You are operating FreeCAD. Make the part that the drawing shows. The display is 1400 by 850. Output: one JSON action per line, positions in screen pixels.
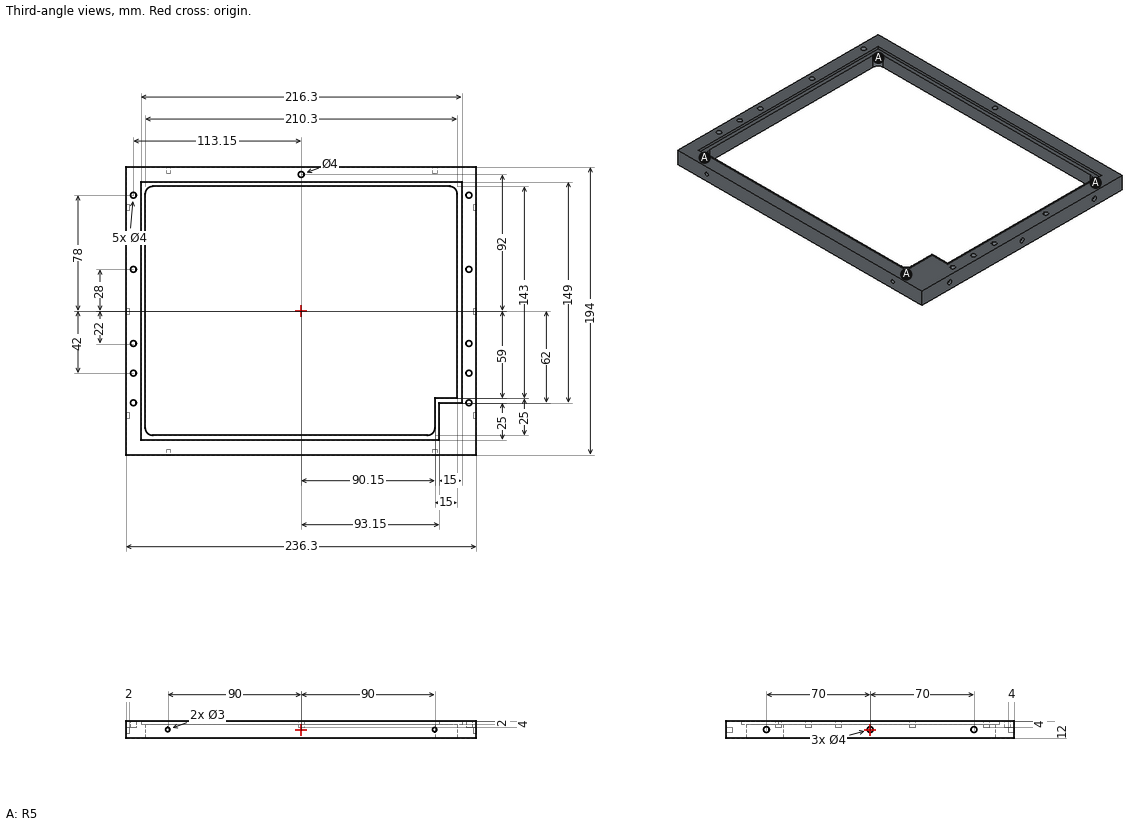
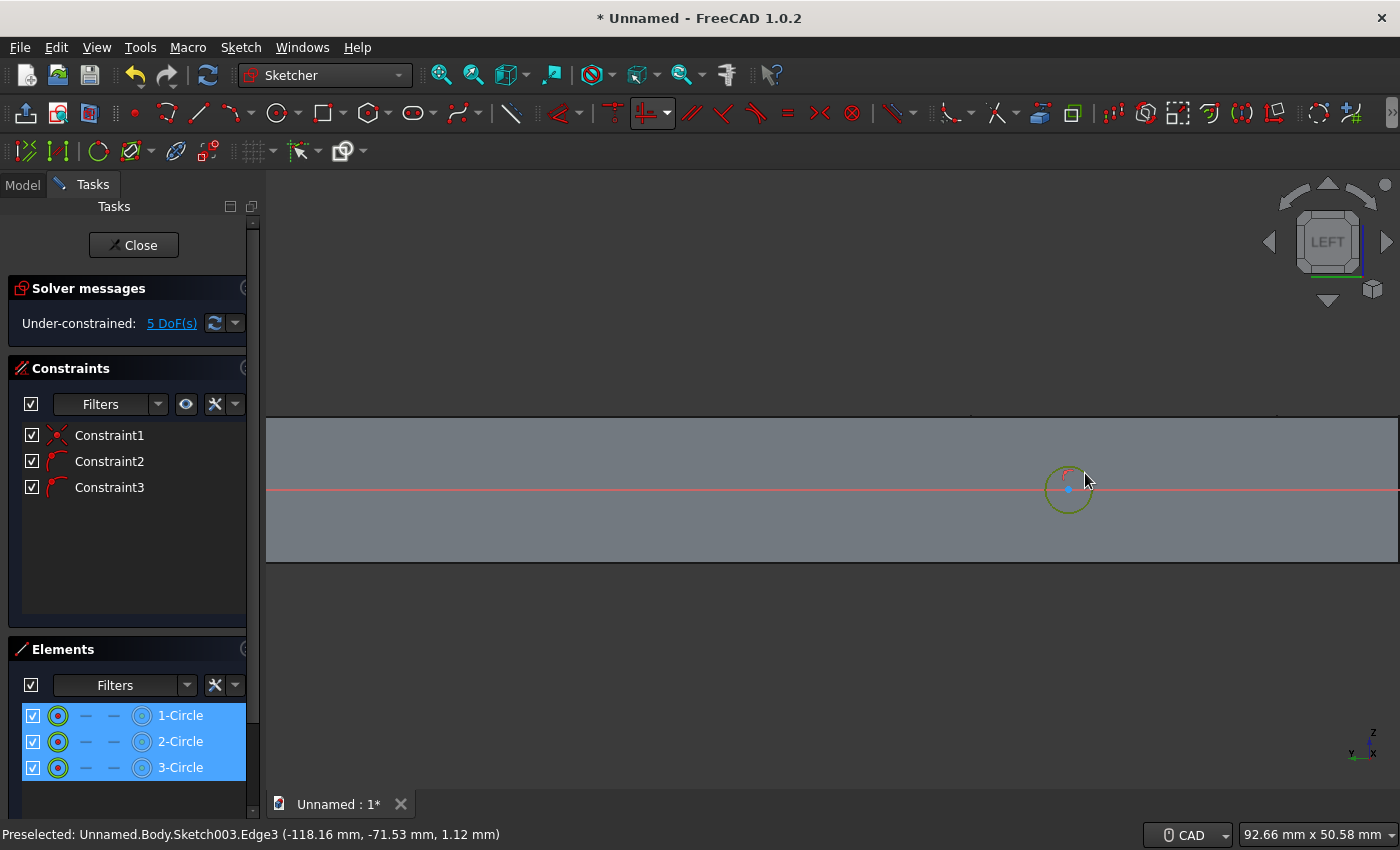
{"action": "left_click", "coordinate": [788, 114]}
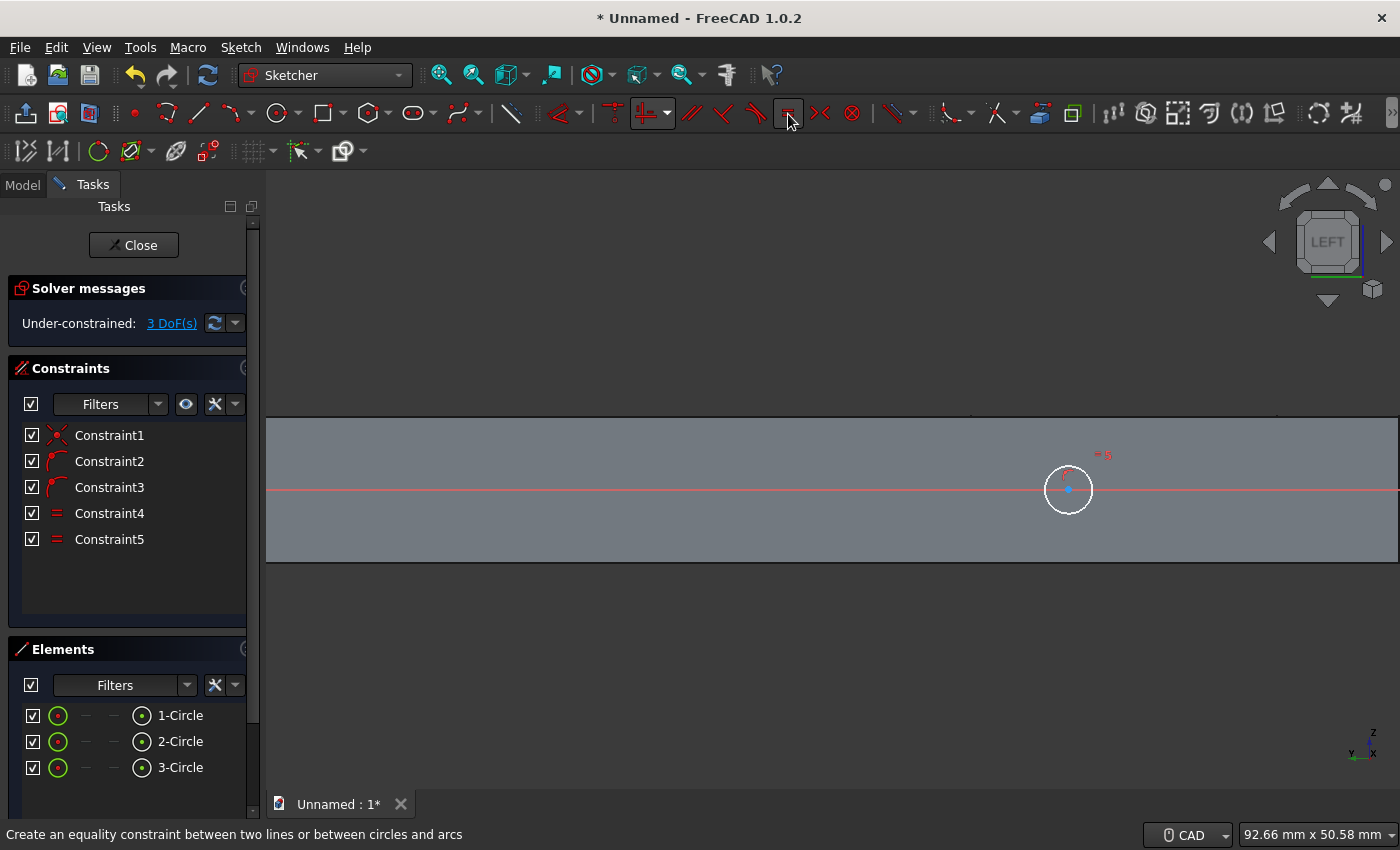
{"action": "left_click", "coordinate": [558, 114]}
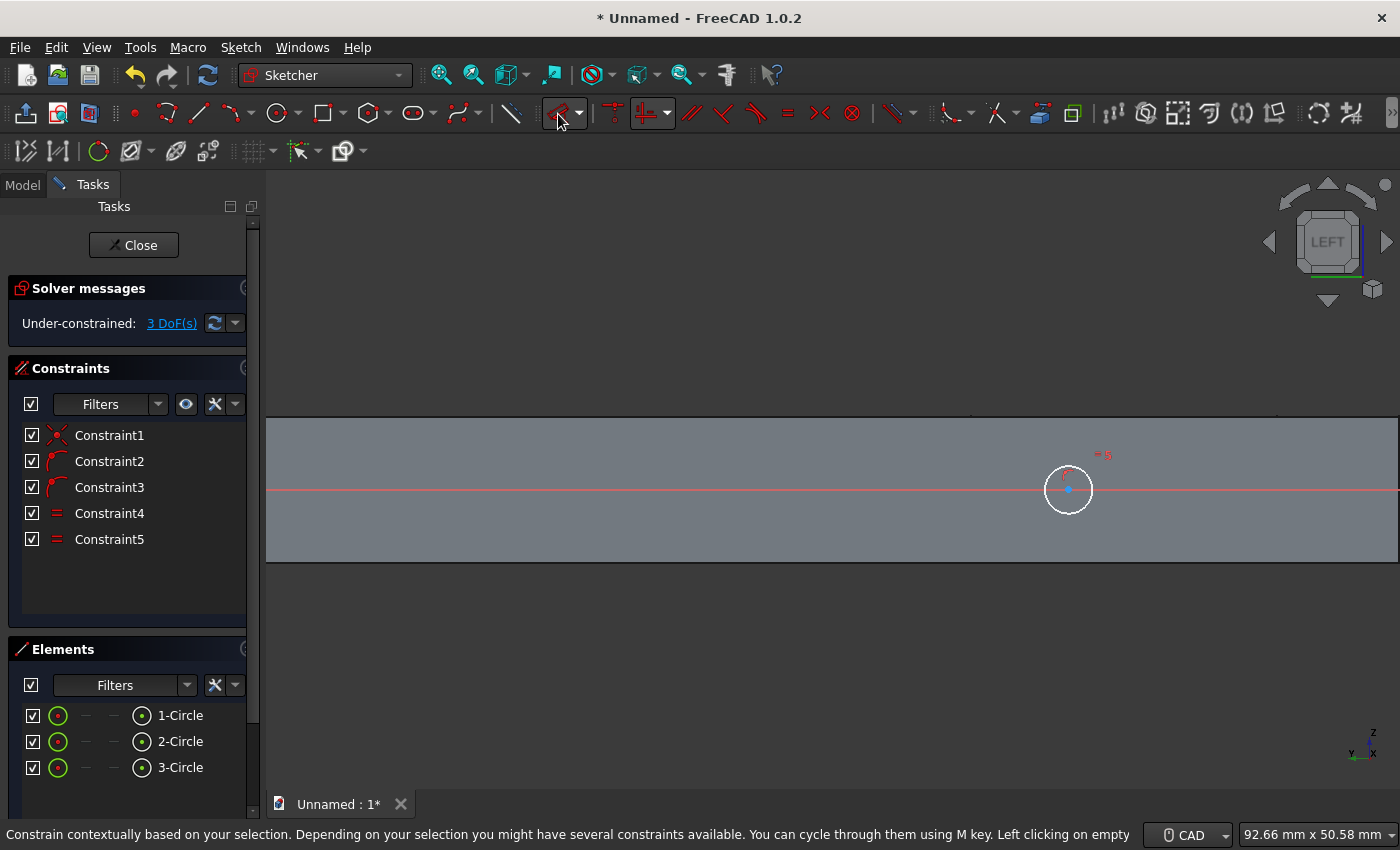
{"action": "scroll", "coordinate": [1086, 473], "scroll_direction": "down", "scroll_amount": 5}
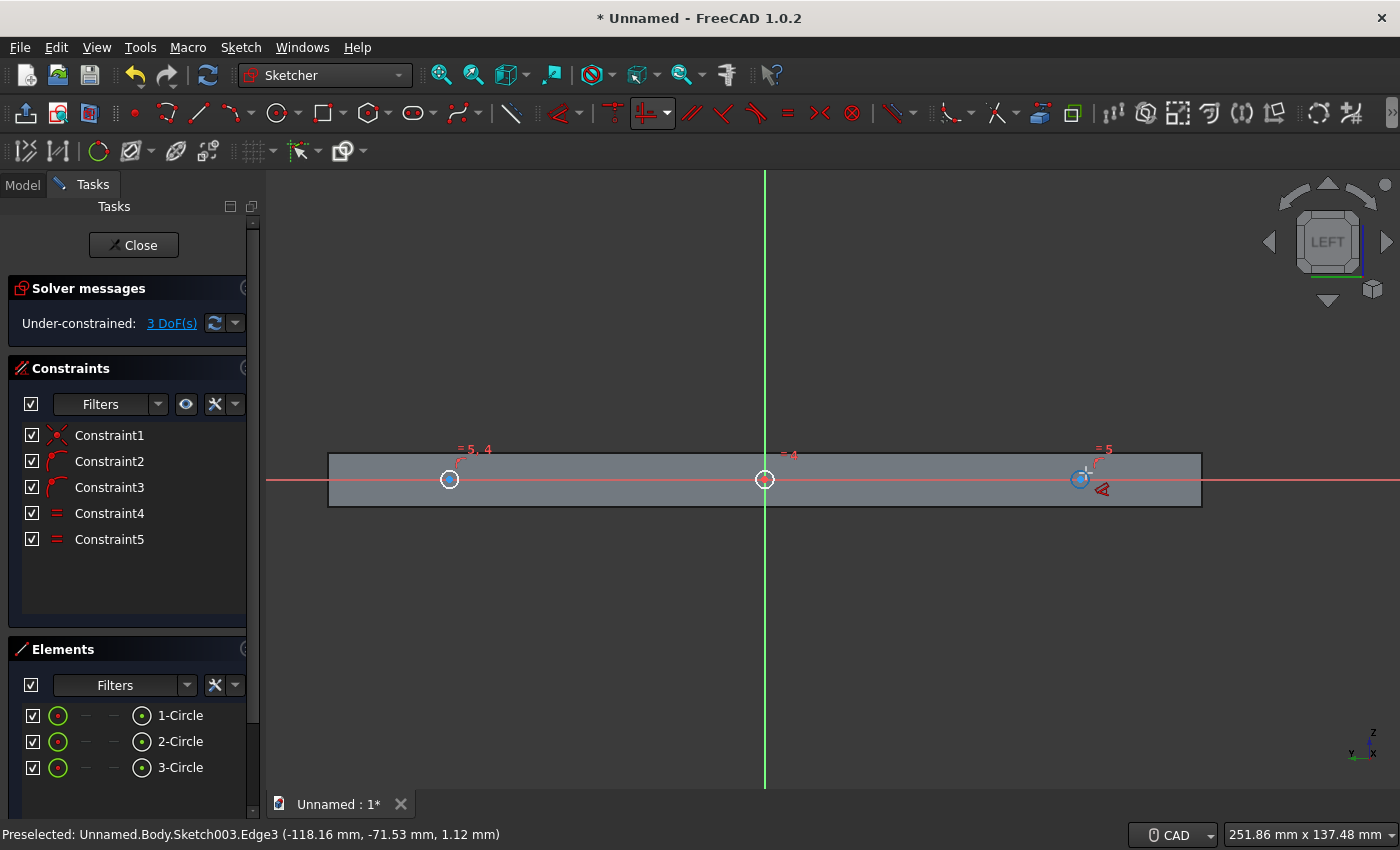
{"action": "scroll", "coordinate": [771, 473], "scroll_direction": "up", "scroll_amount": 5}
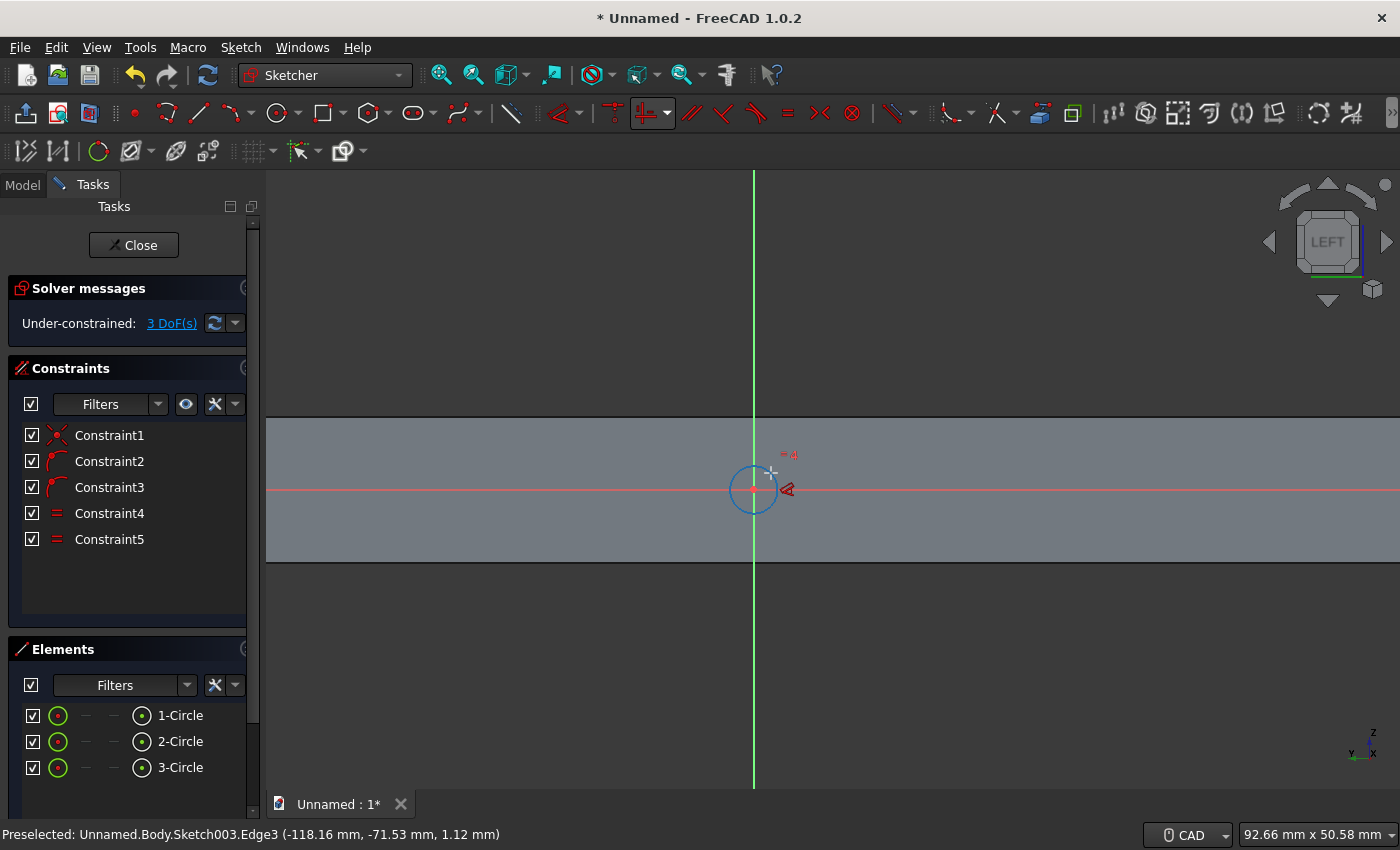
{"action": "left_click", "coordinate": [771, 473]}
{"action": "left_click", "coordinate": [794, 451]}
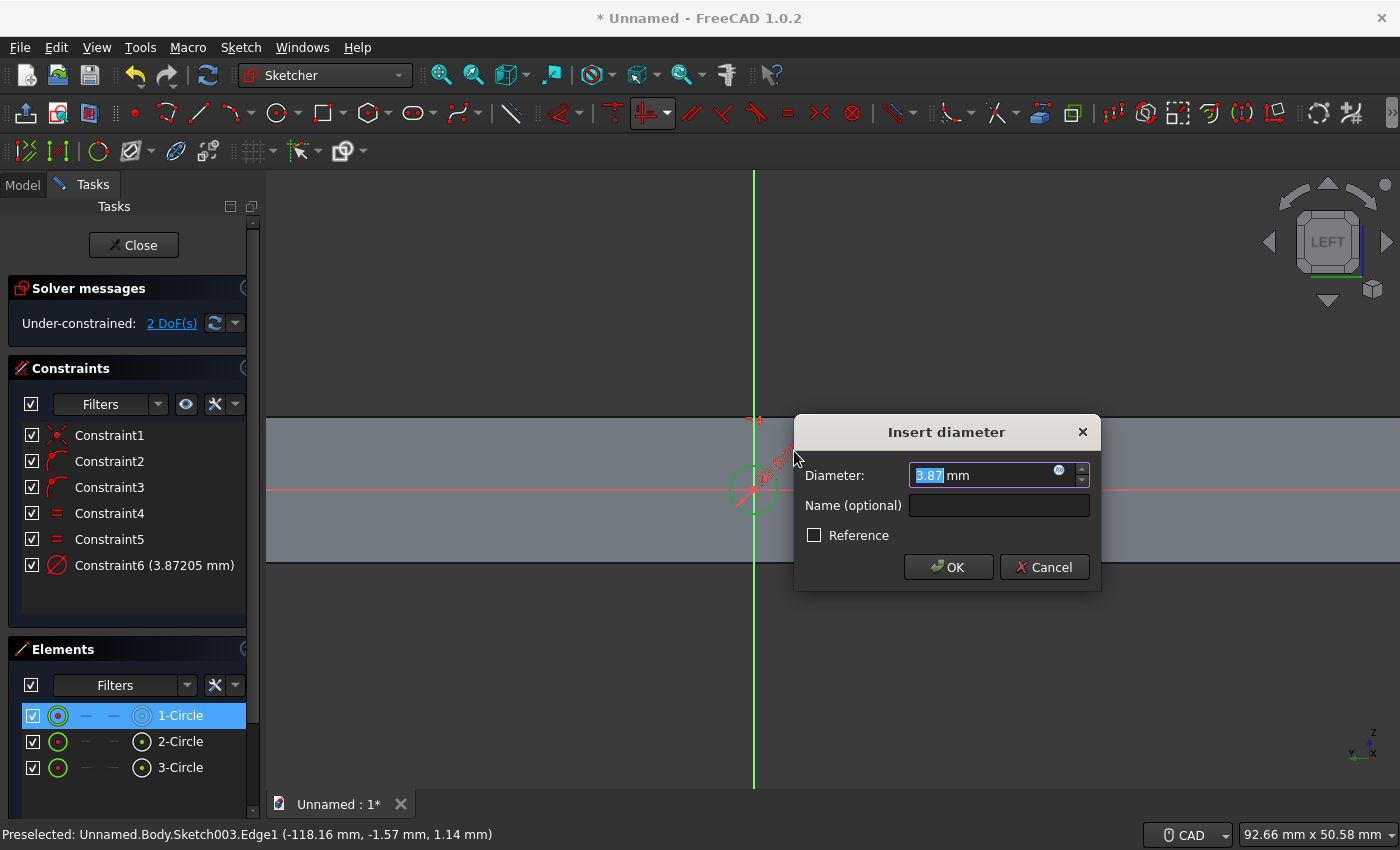
{"action": "type", "text": "4"}
{"action": "key", "text": "Return"}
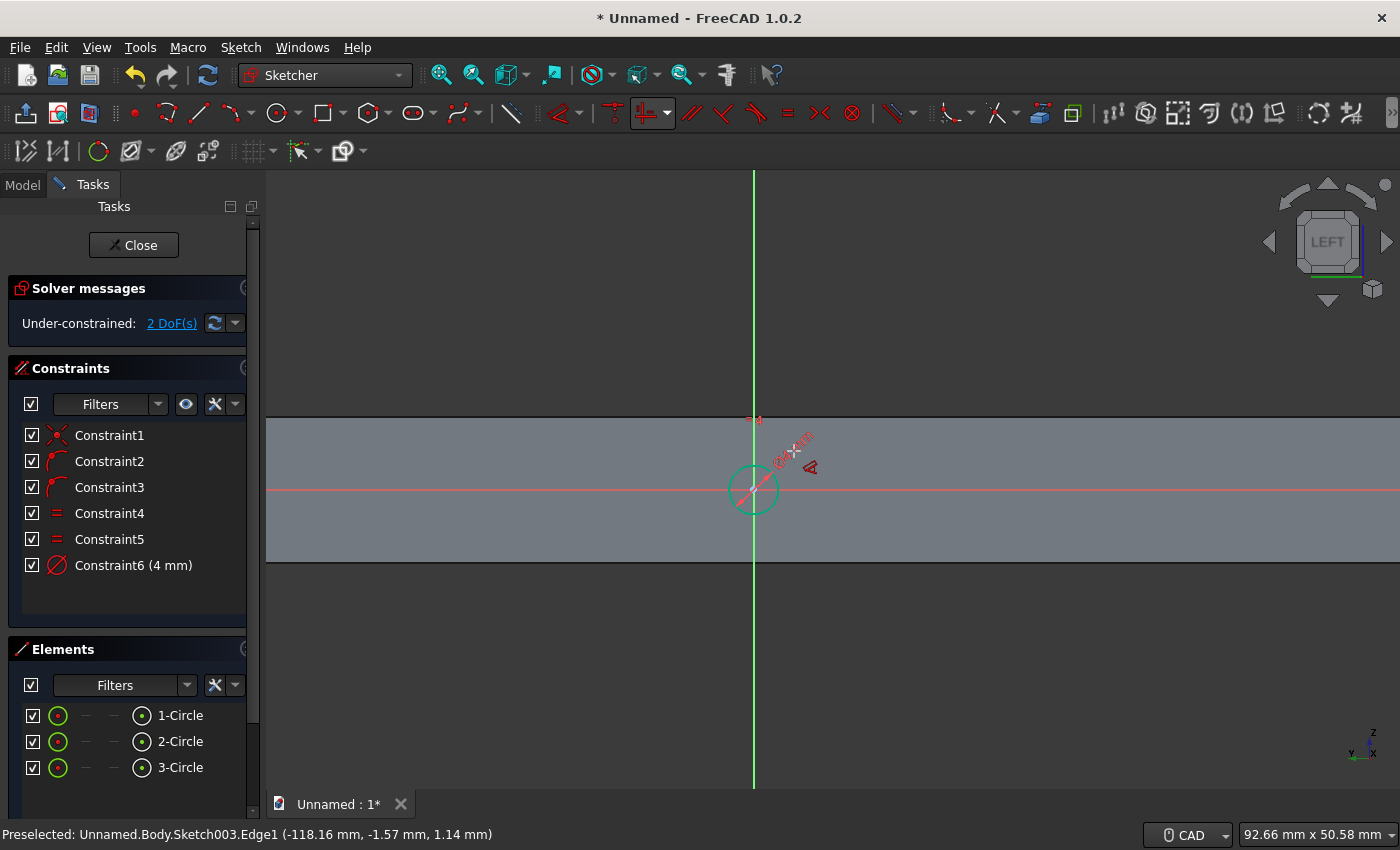
{"action": "scroll", "coordinate": [771, 473], "scroll_direction": "down", "scroll_amount": 5}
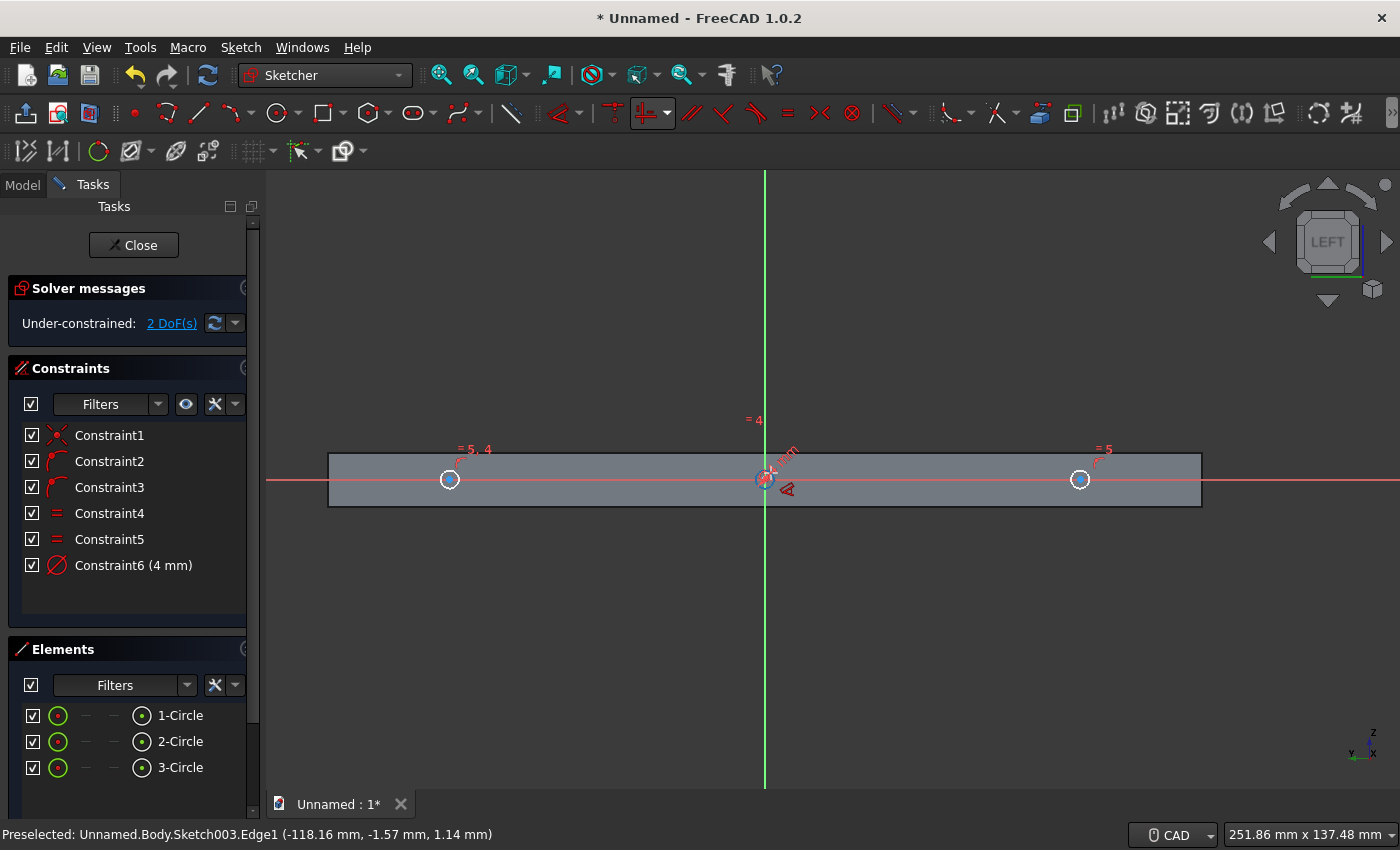
{"action": "left_click", "coordinate": [450, 480]}
{"action": "left_click", "coordinate": [607, 514]}